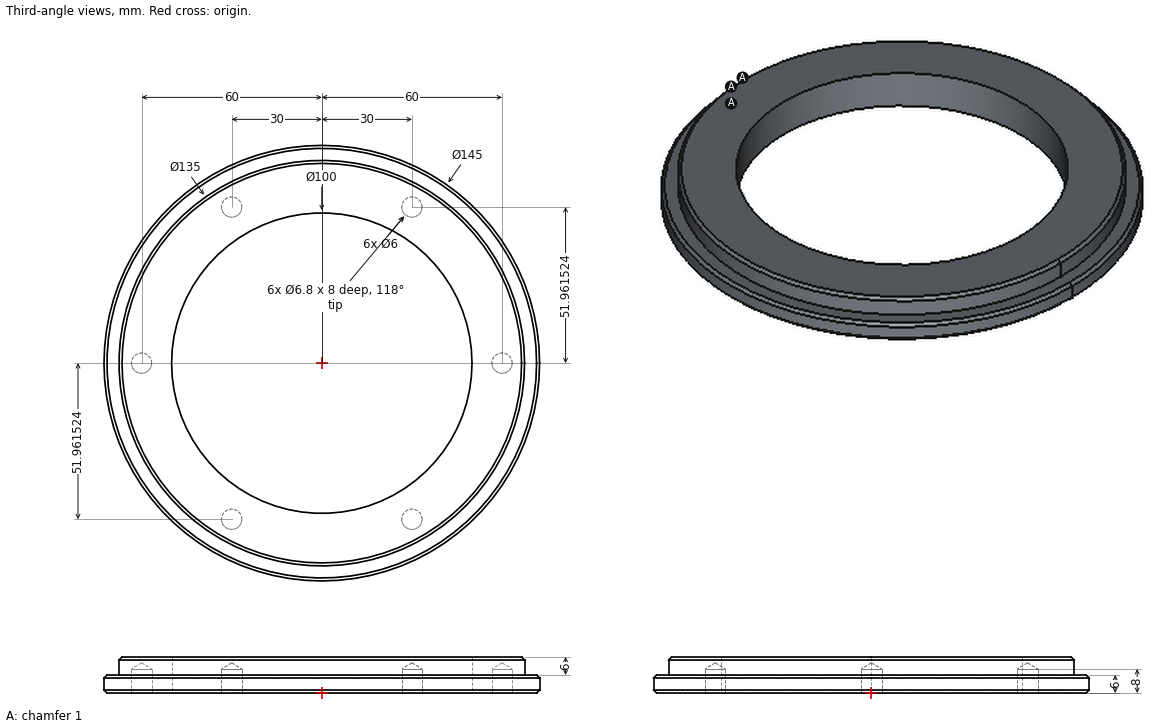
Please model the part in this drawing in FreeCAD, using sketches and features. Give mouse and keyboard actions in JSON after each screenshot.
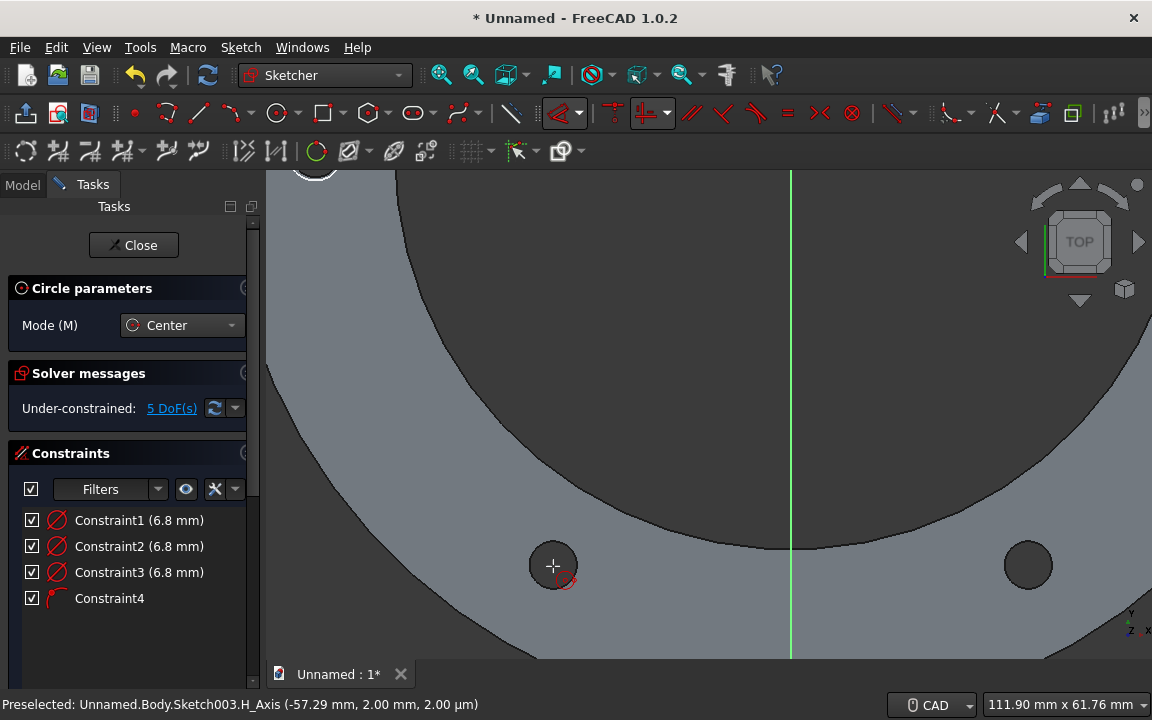
{"action": "left_click", "coordinate": [553, 565]}
{"action": "mouse_move", "coordinate": [572, 546]}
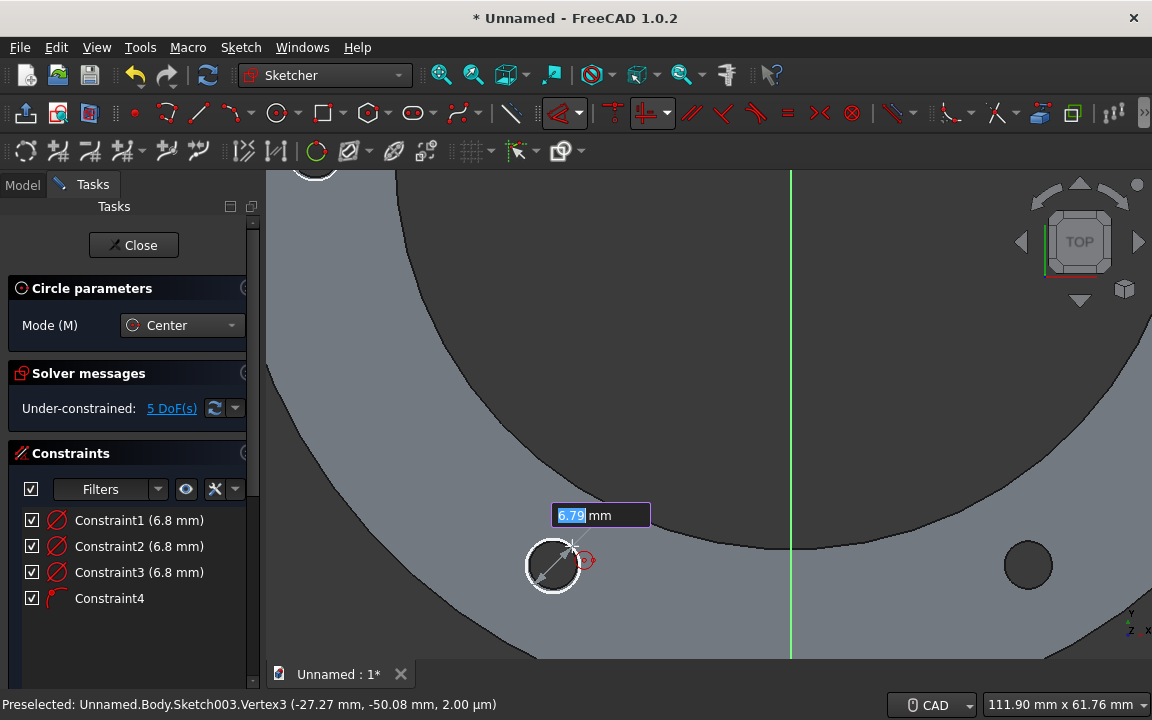
{"action": "type", "text": "6.8"}
{"action": "key", "text": "Return"}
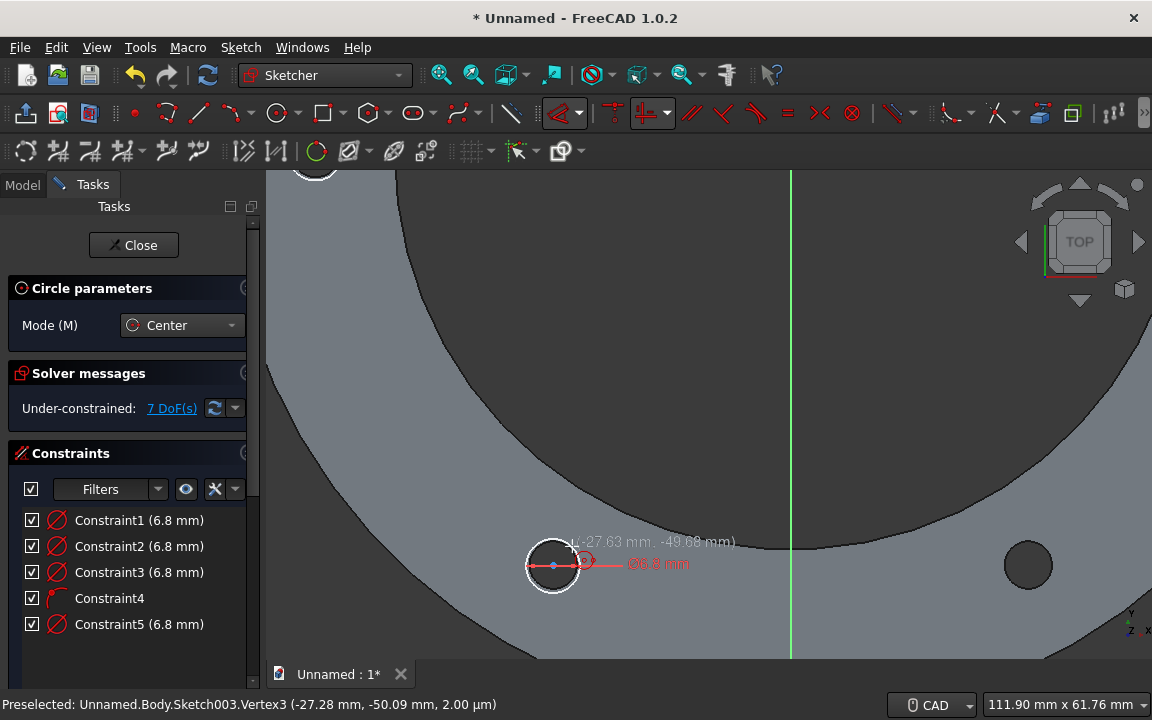
{"action": "scroll", "coordinate": [553, 566], "scroll_direction": "down", "scroll_amount": 5}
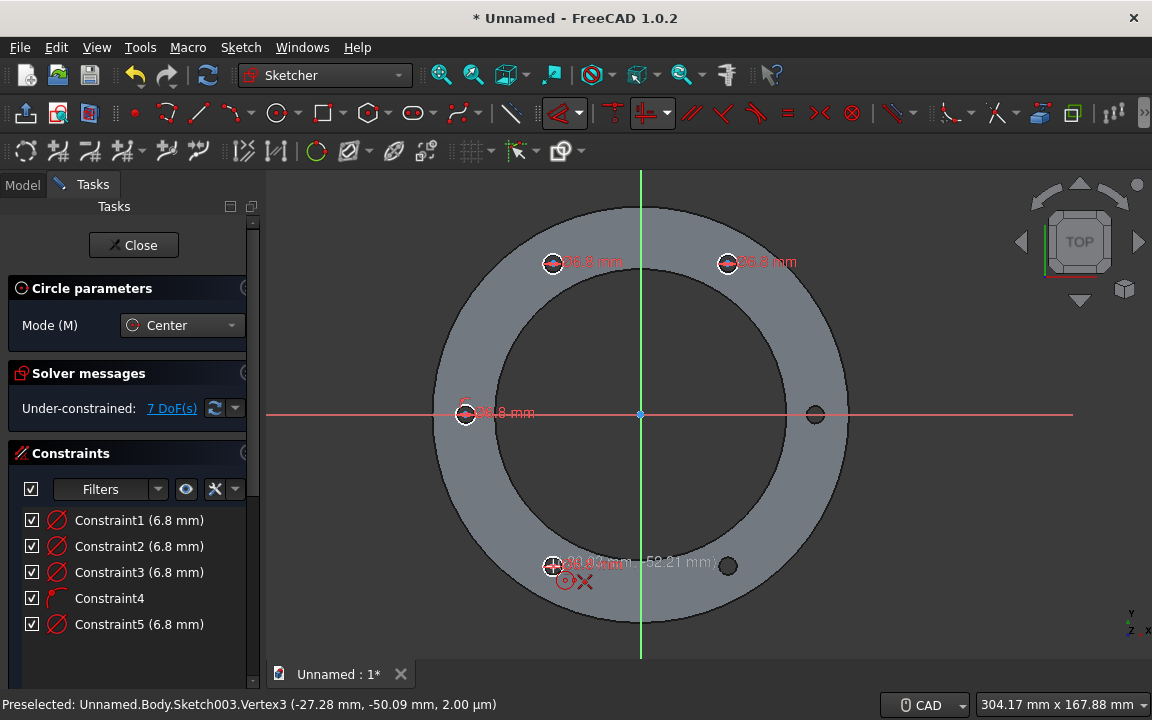
{"action": "scroll", "coordinate": [728, 566], "scroll_direction": "up", "scroll_amount": 5}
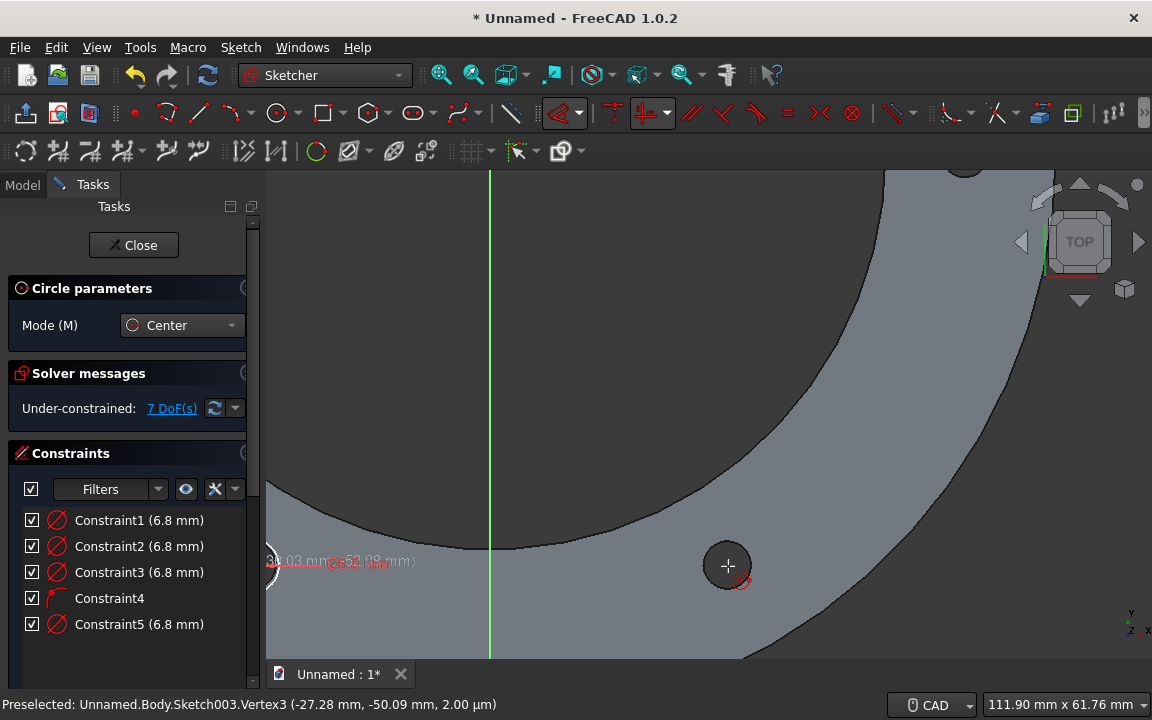
{"action": "left_click", "coordinate": [727, 565]}
{"action": "mouse_move", "coordinate": [746, 546]}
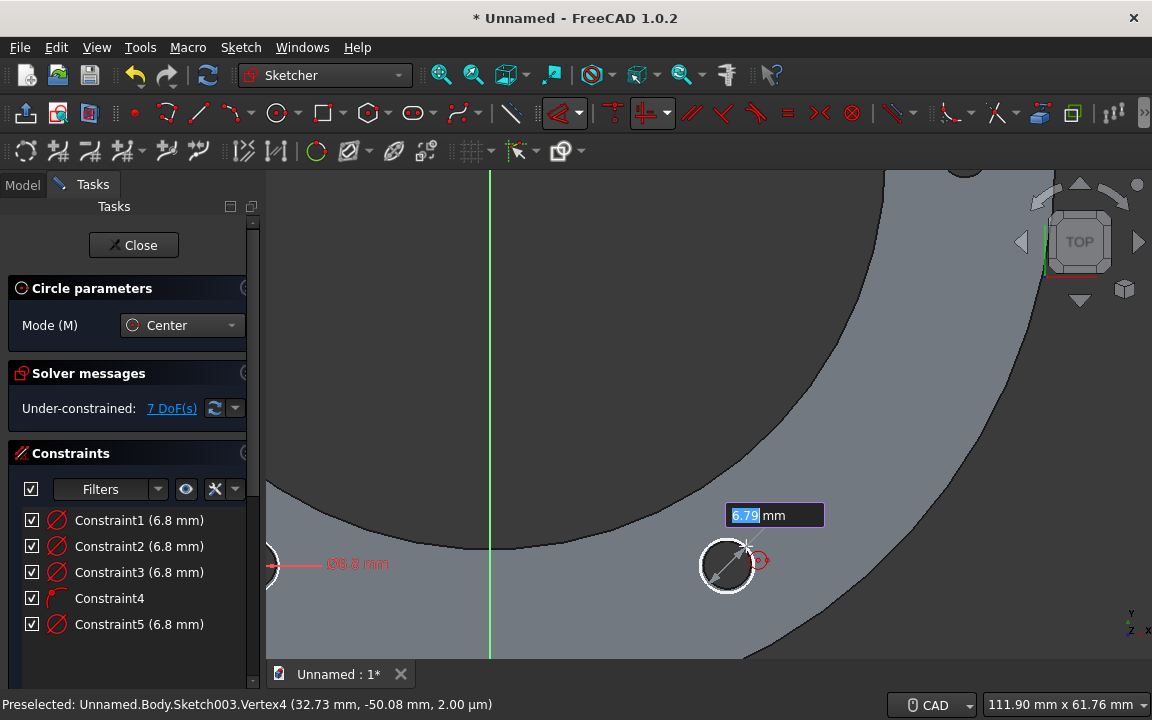
{"action": "type", "text": "6.8"}
{"action": "key", "text": "Return"}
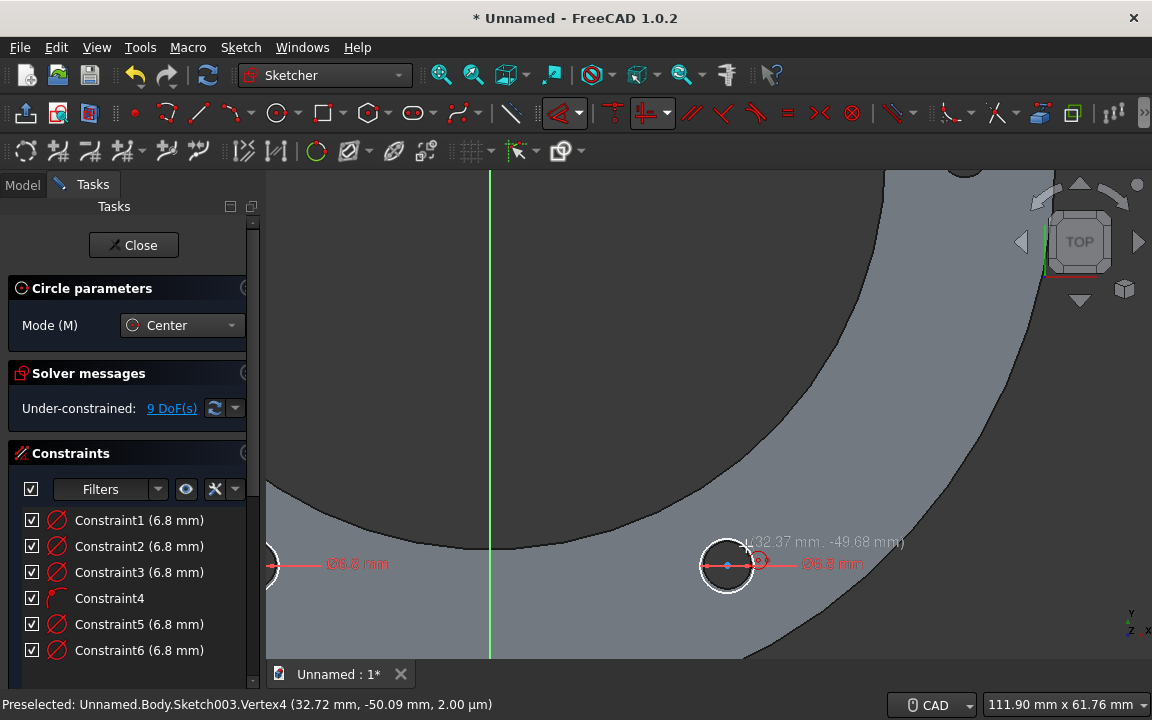
{"action": "scroll", "coordinate": [728, 566], "scroll_direction": "down", "scroll_amount": 5}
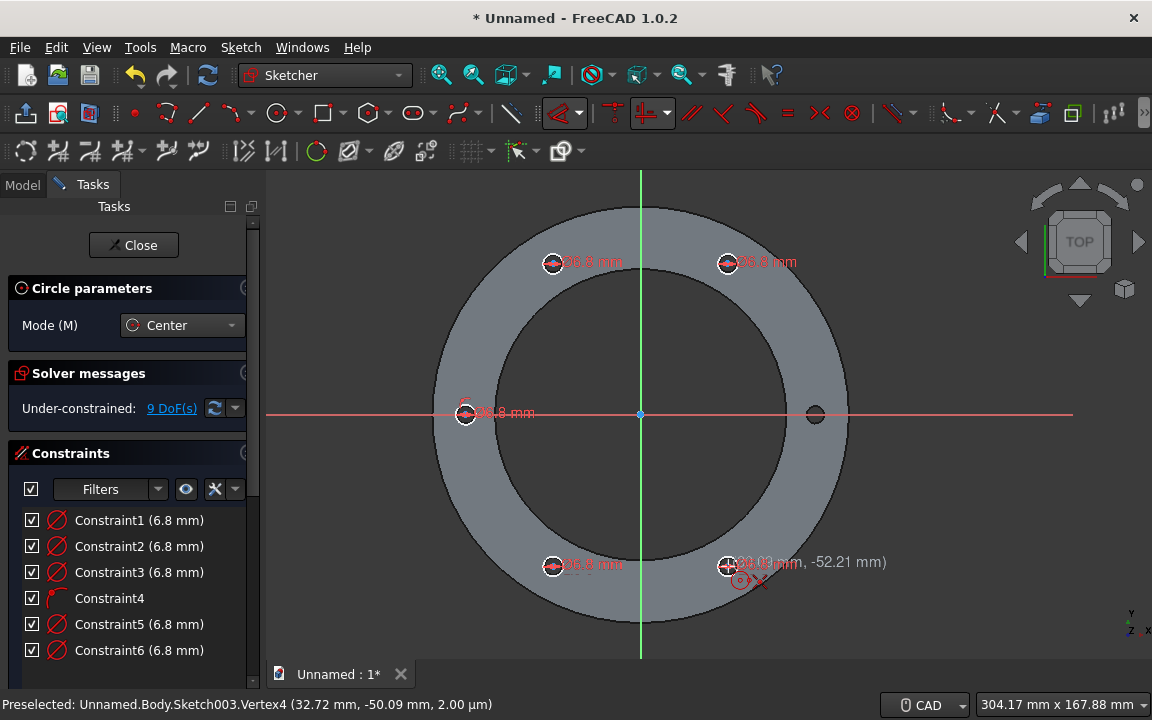
{"action": "scroll", "coordinate": [815, 415], "scroll_direction": "up", "scroll_amount": 5}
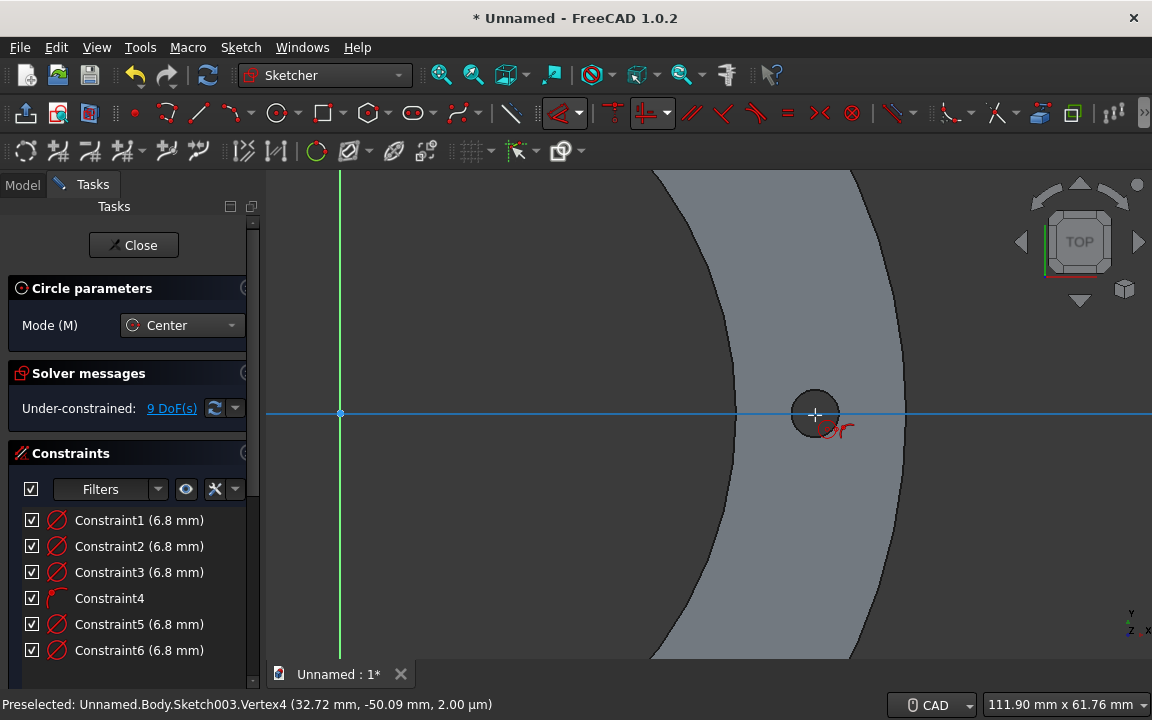
{"action": "left_click", "coordinate": [815, 414]}
{"action": "mouse_move", "coordinate": [834, 395]}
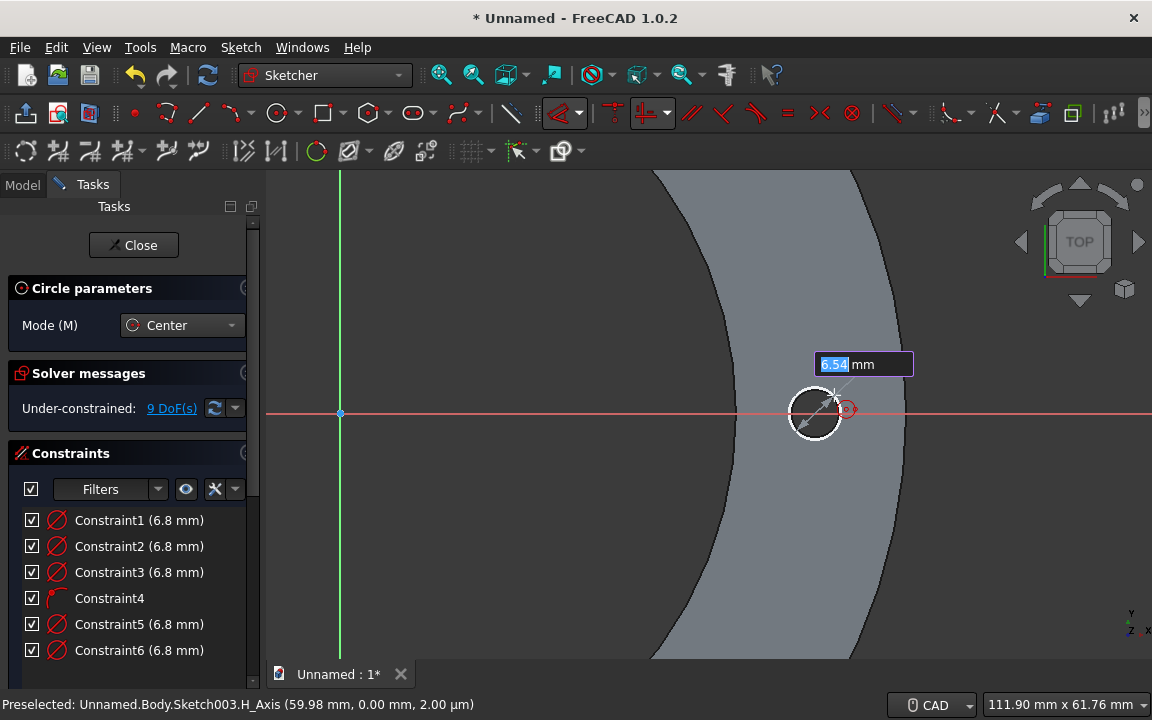
{"action": "type", "text": "6.8"}
{"action": "key", "text": "Return"}
{"action": "key", "text": "Escape"}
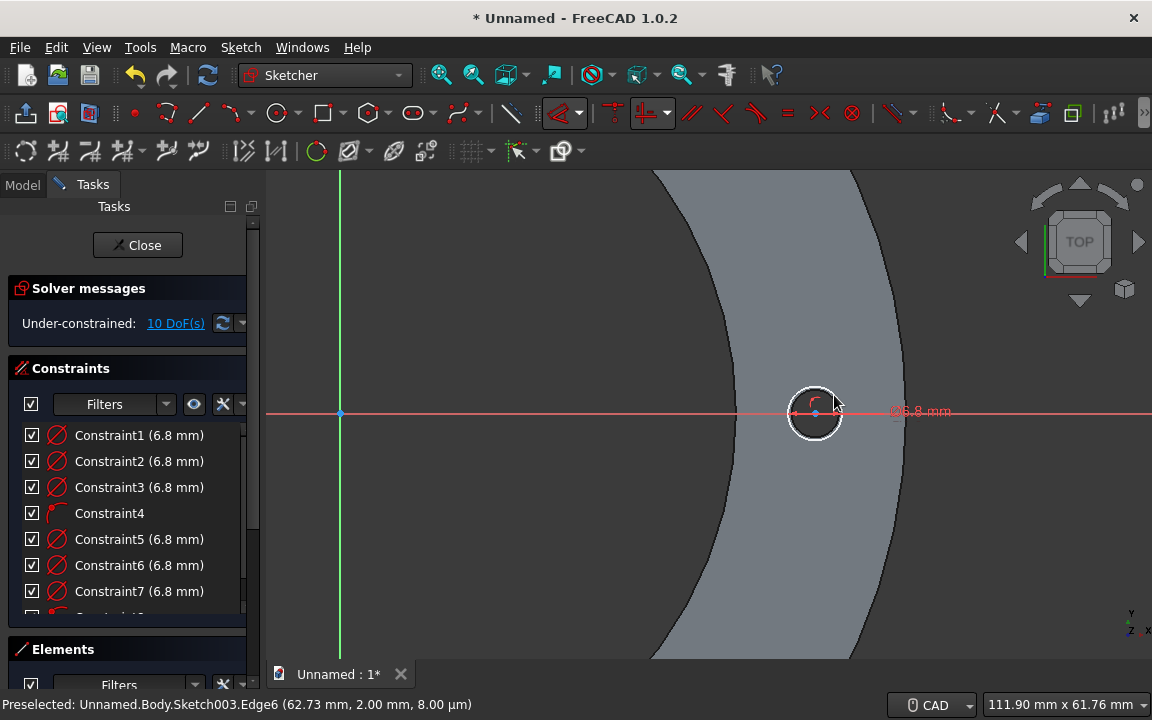
{"action": "scroll", "coordinate": [815, 415], "scroll_direction": "down", "scroll_amount": 5}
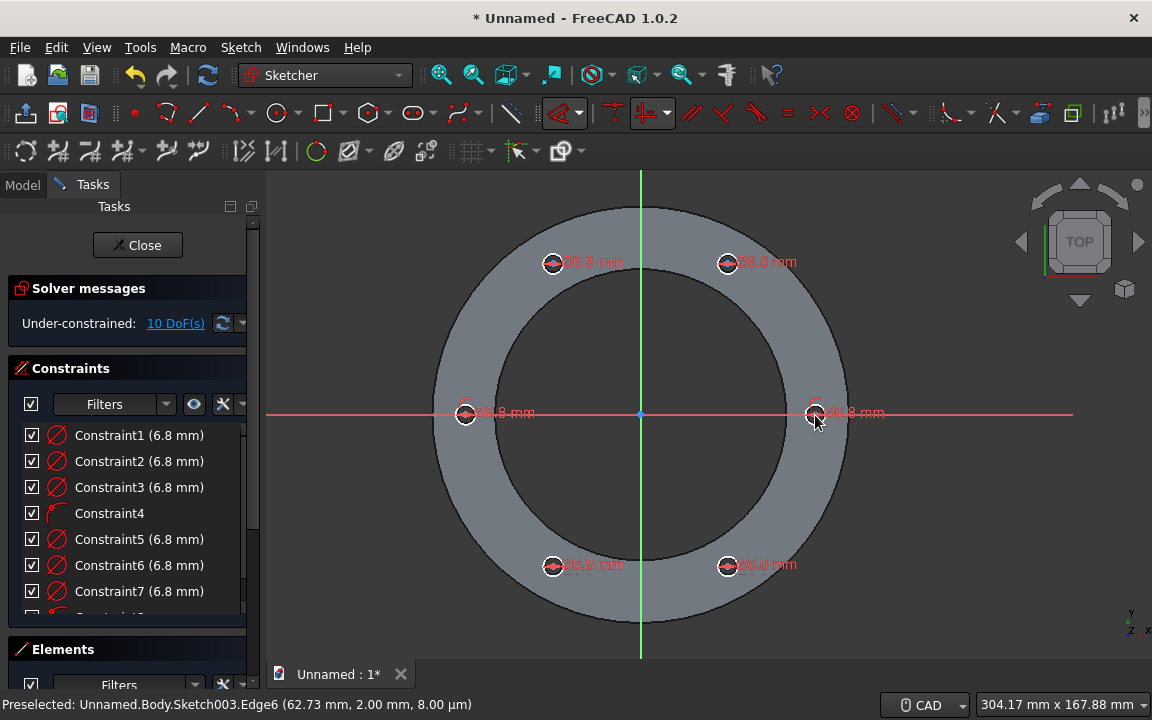
{"action": "left_click", "coordinate": [728, 264]}